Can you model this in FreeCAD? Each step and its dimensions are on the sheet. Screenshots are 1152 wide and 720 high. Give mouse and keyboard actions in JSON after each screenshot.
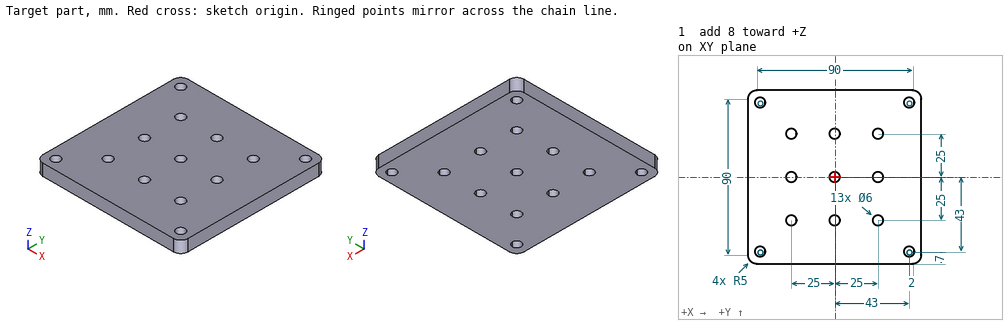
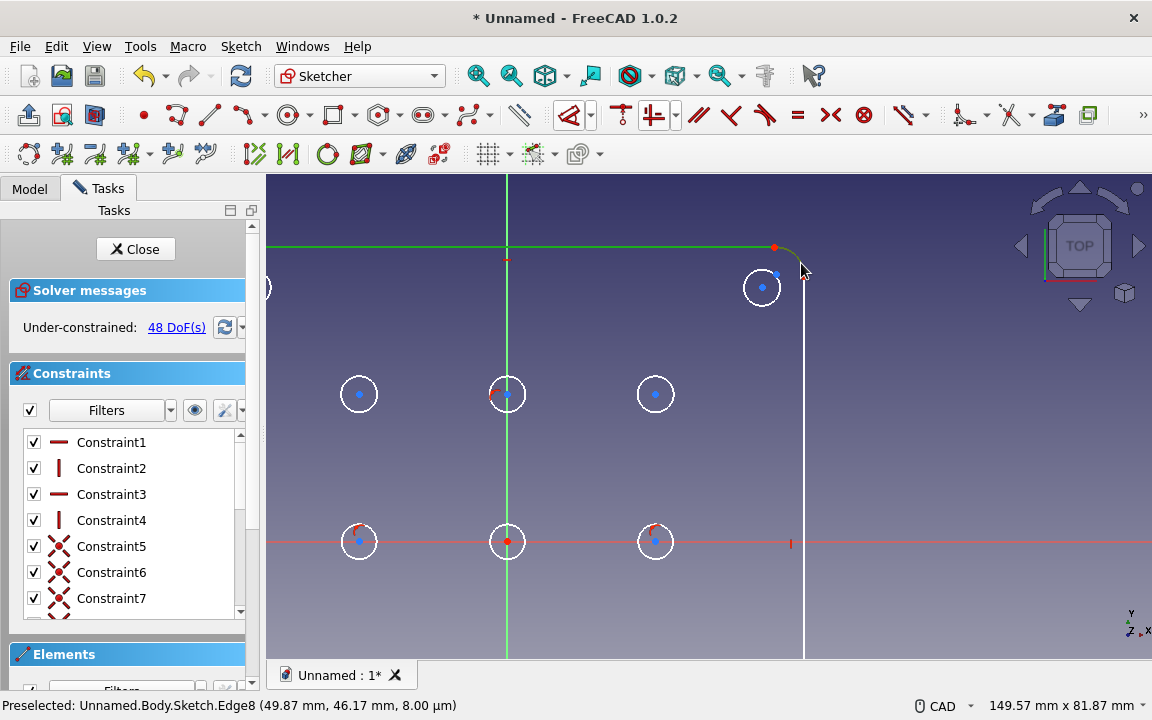
{"action": "left_click", "coordinate": [765, 116]}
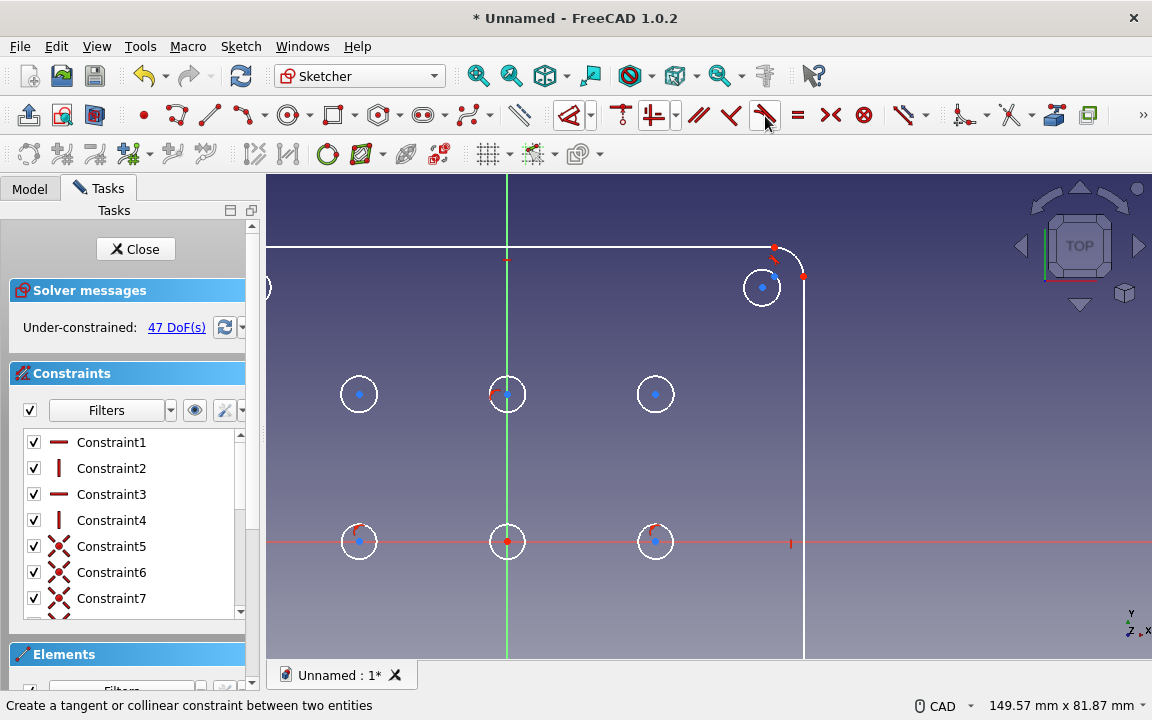
{"action": "scroll", "coordinate": [802, 264], "scroll_direction": "down", "scroll_amount": 3}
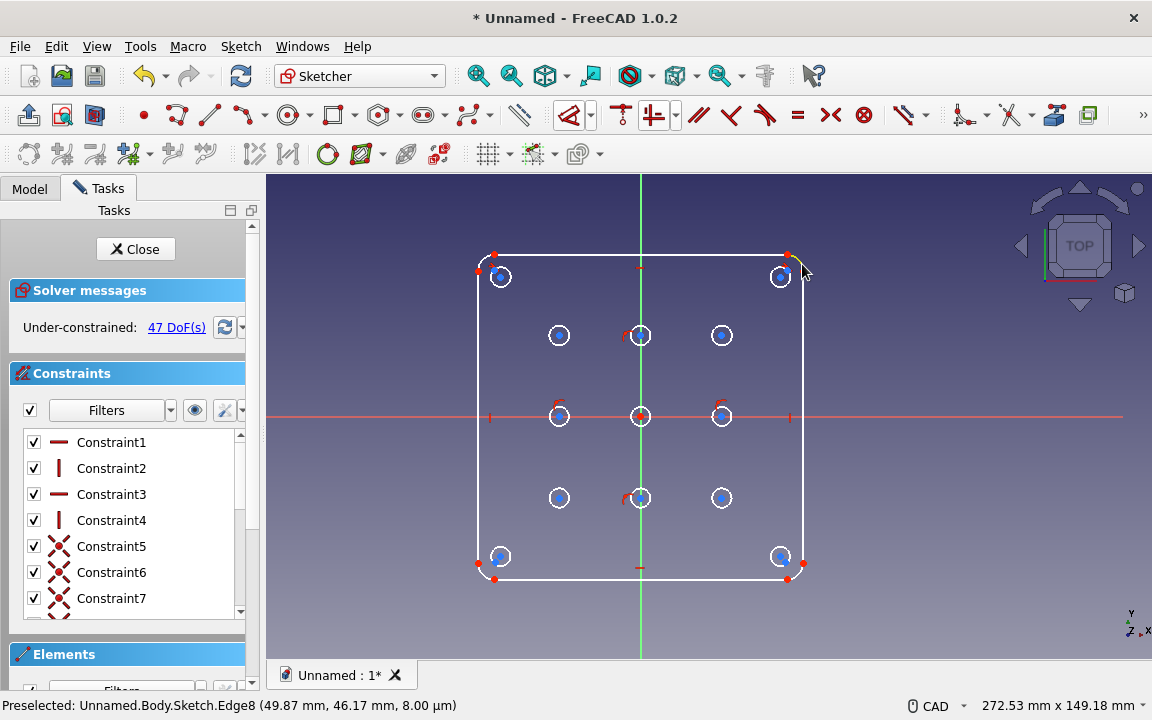
{"action": "left_click", "coordinate": [478, 359]}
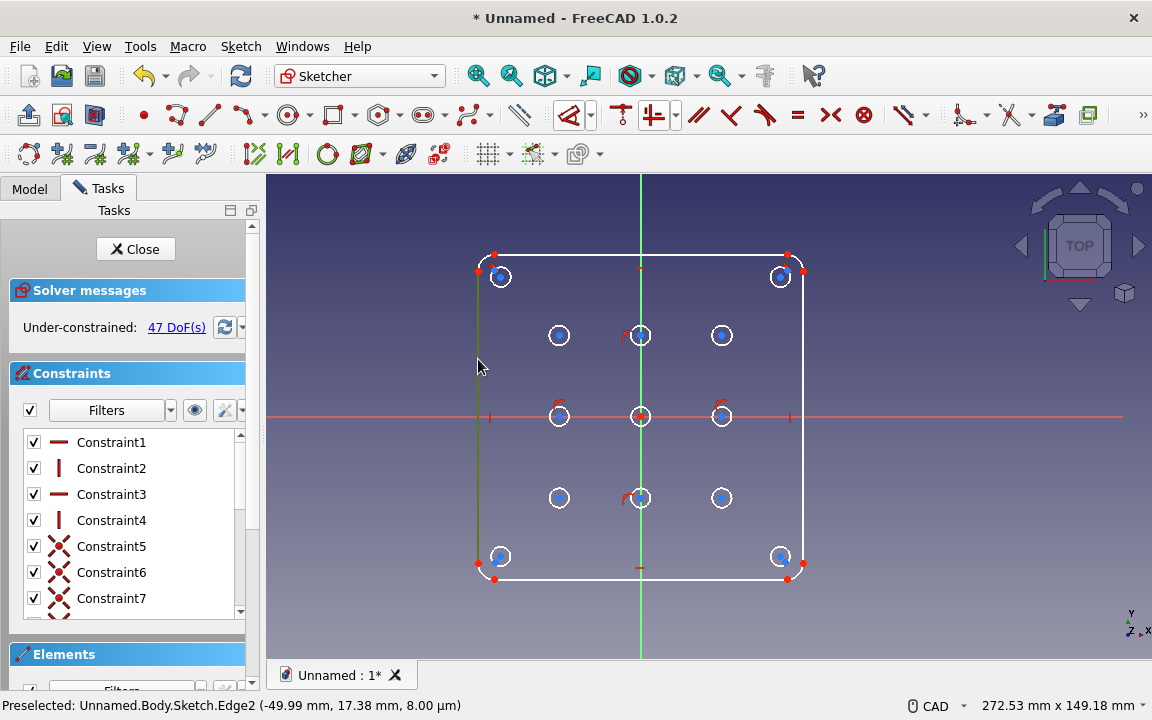
{"action": "left_click", "coordinate": [483, 260]}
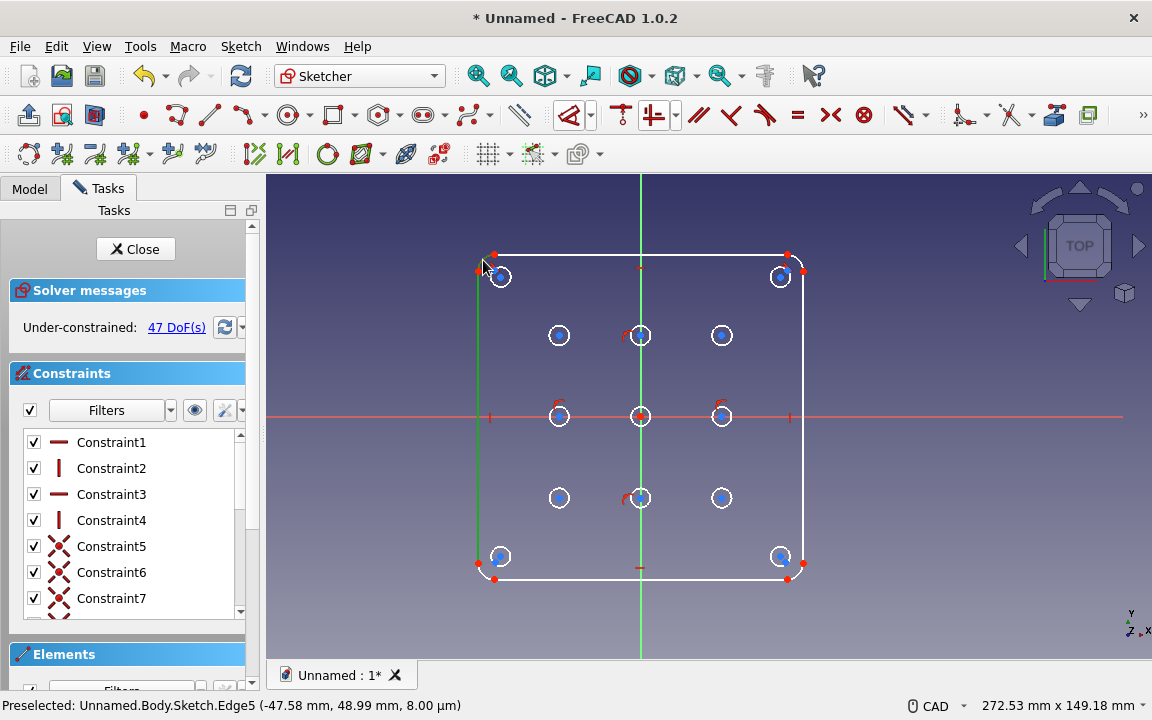
{"action": "left_click", "coordinate": [765, 116]}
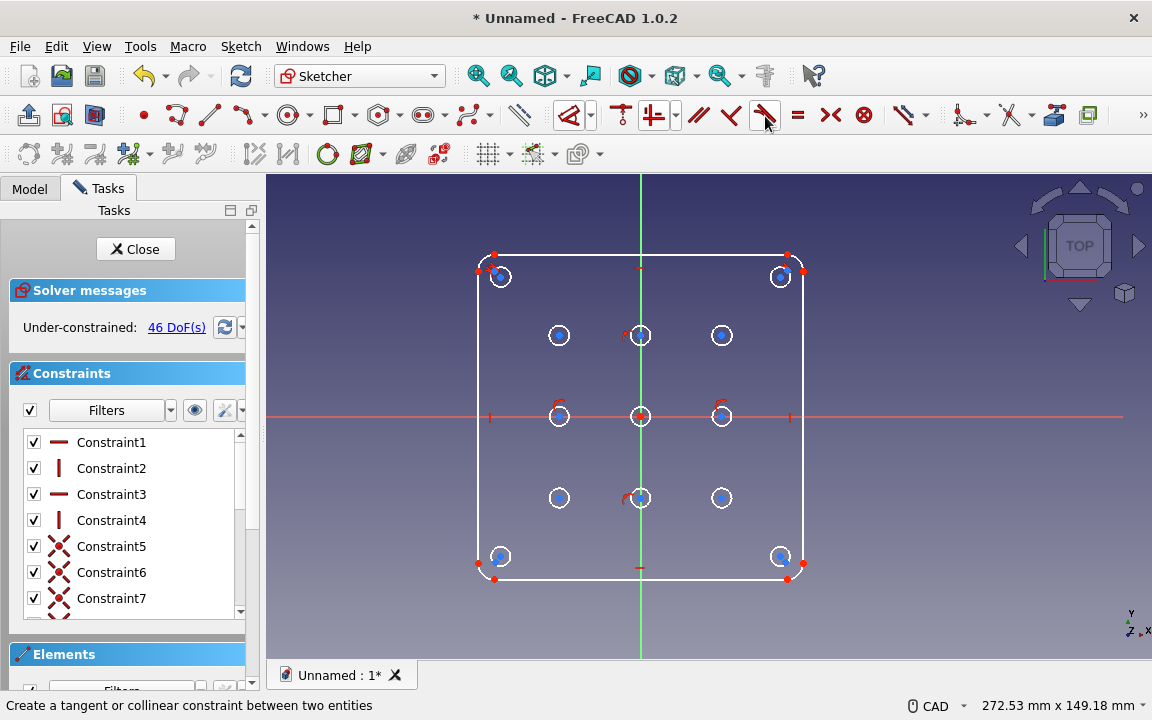
{"action": "left_click", "coordinate": [478, 359]}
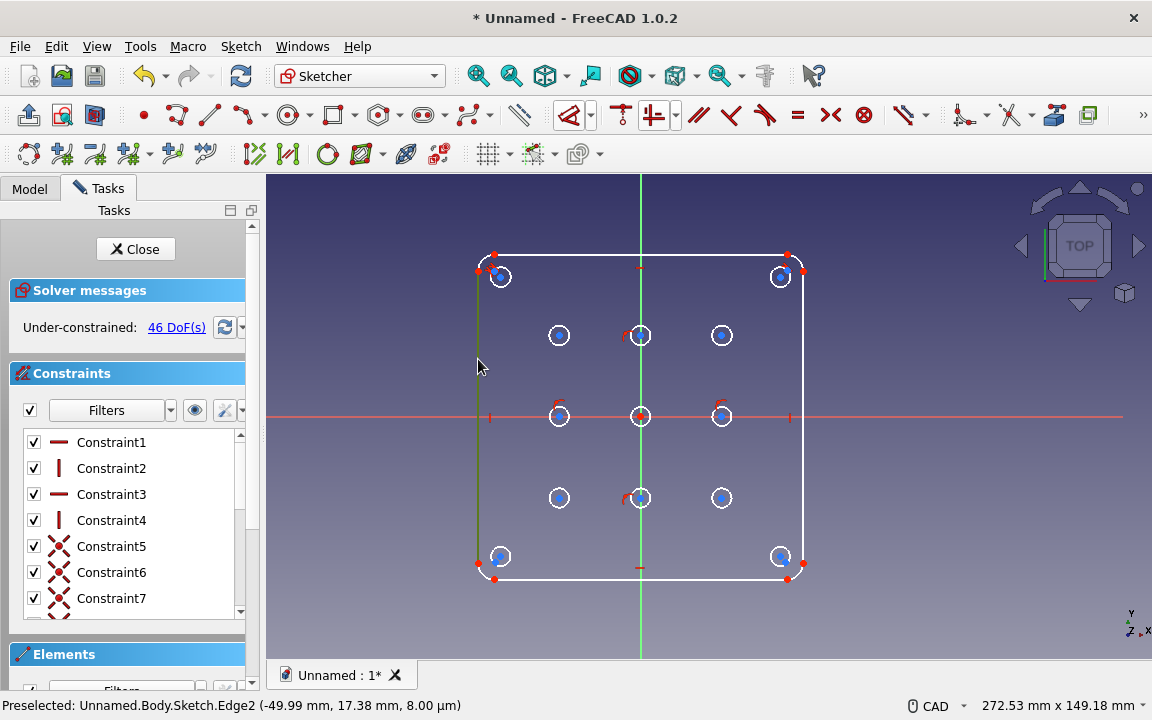
{"action": "left_click", "coordinate": [483, 575]}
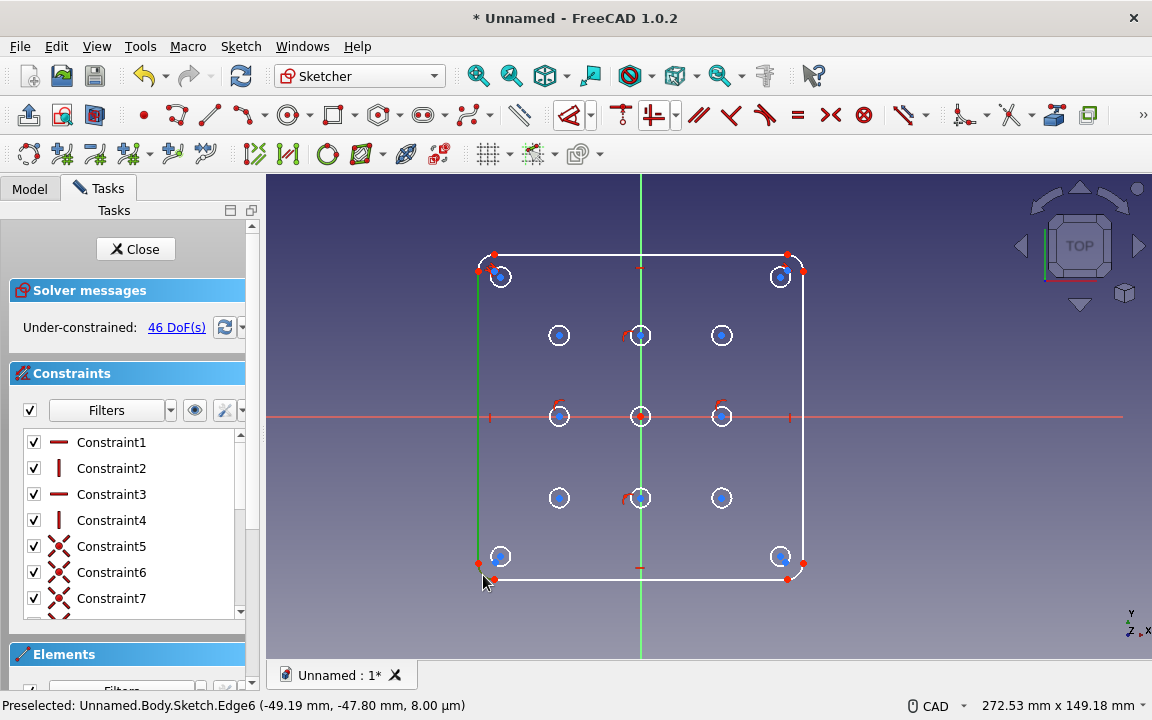
{"action": "left_click", "coordinate": [765, 116]}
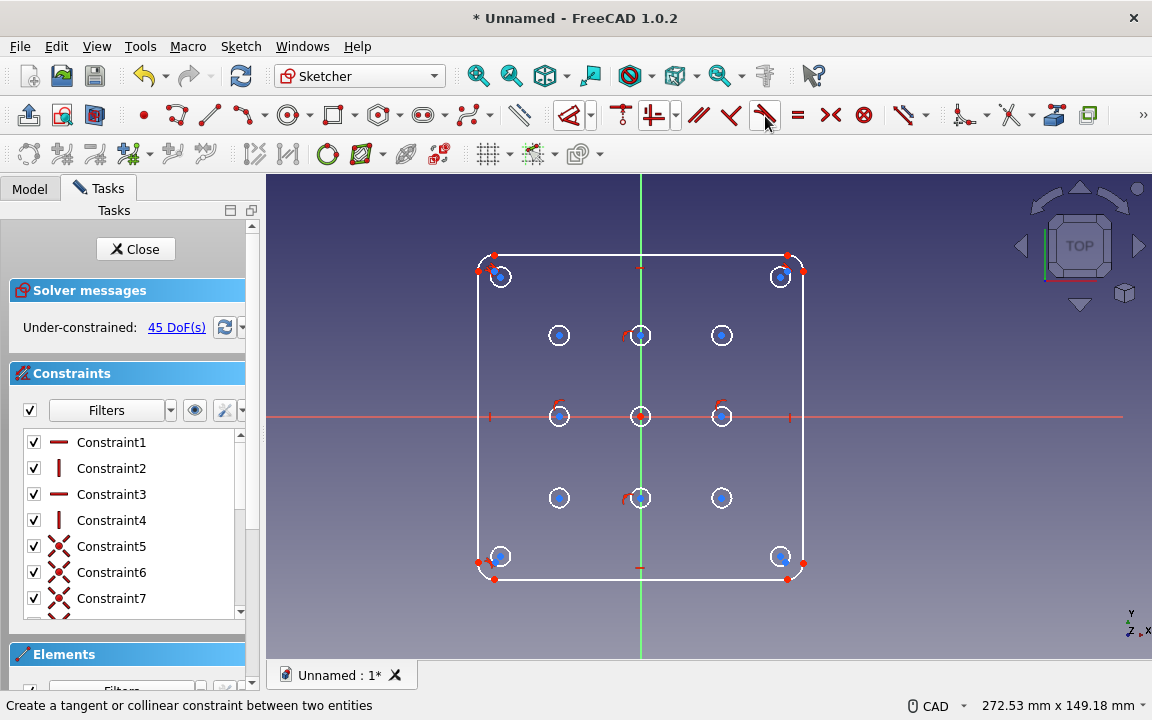
{"action": "left_click", "coordinate": [582, 580]}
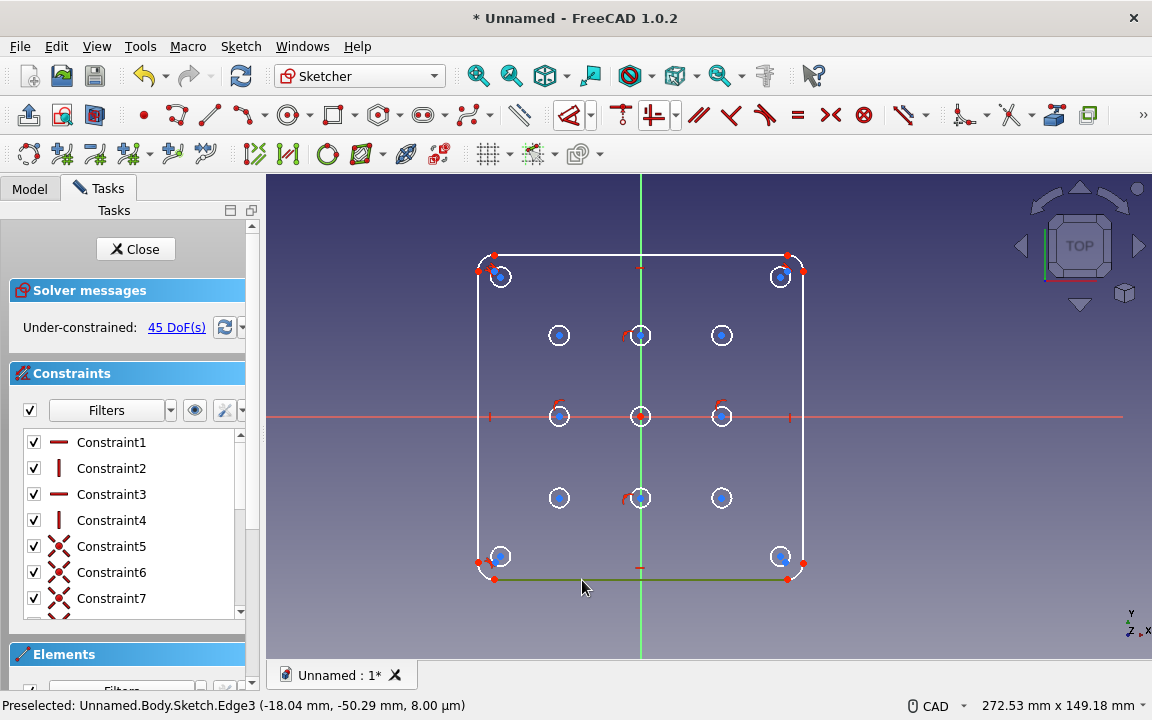
{"action": "left_click", "coordinate": [483, 575]}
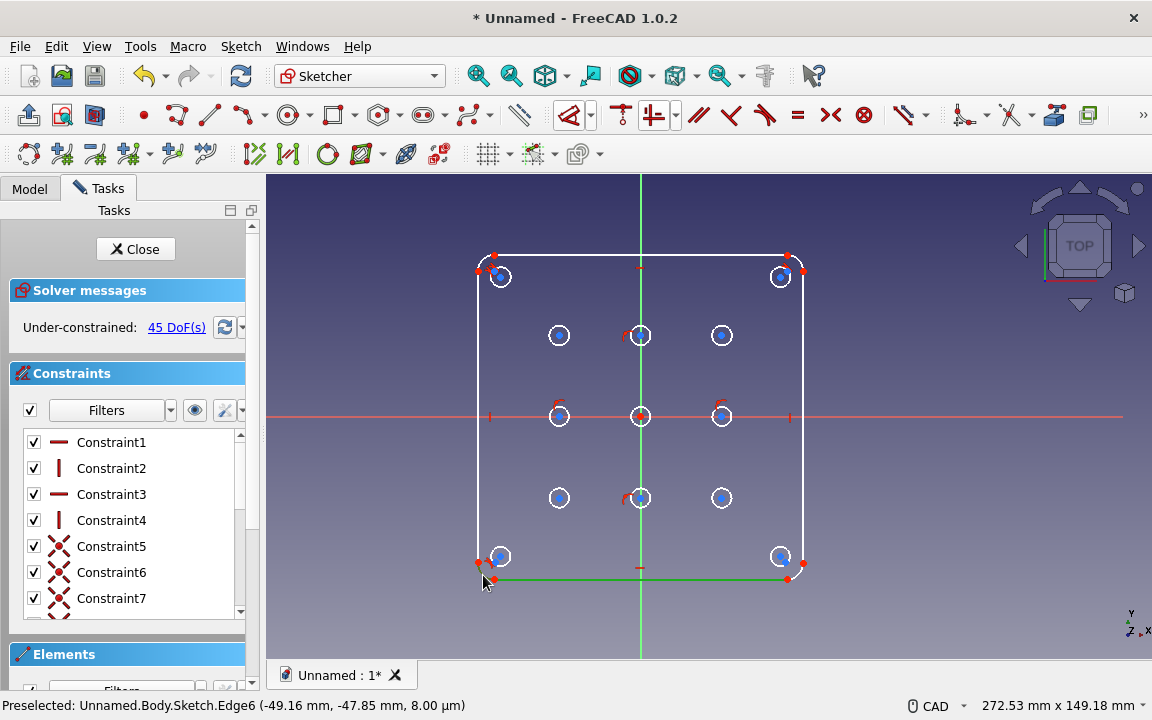
{"action": "left_click", "coordinate": [765, 116]}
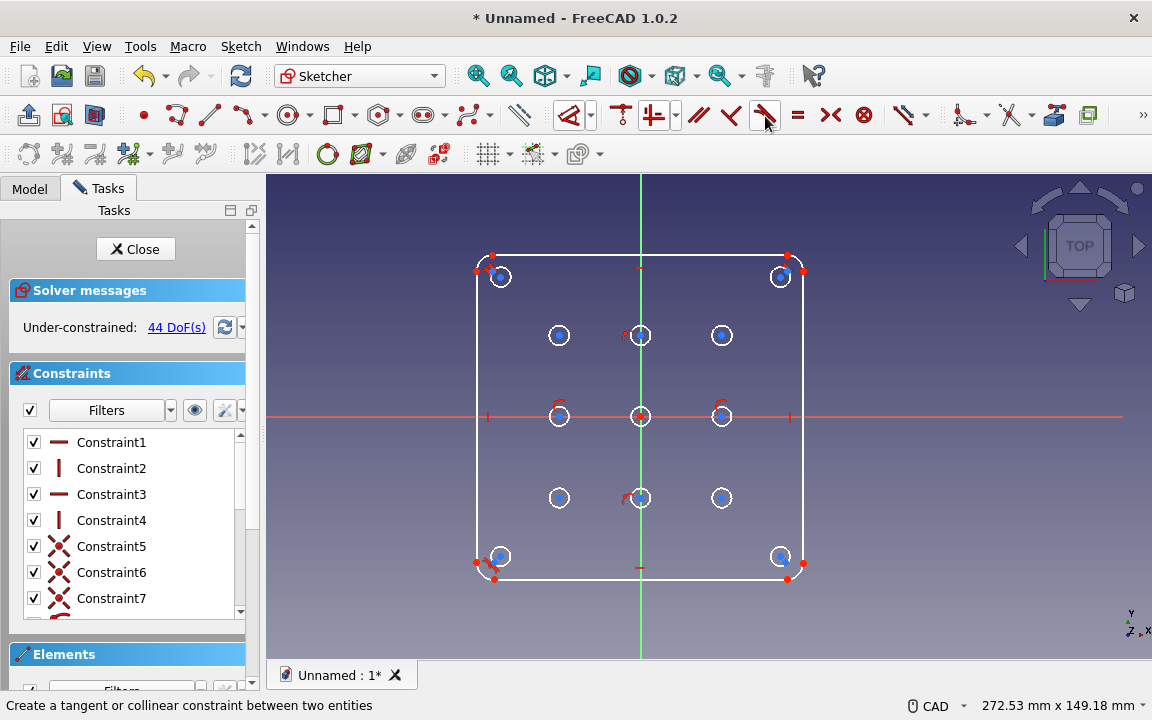
{"action": "left_click", "coordinate": [582, 580]}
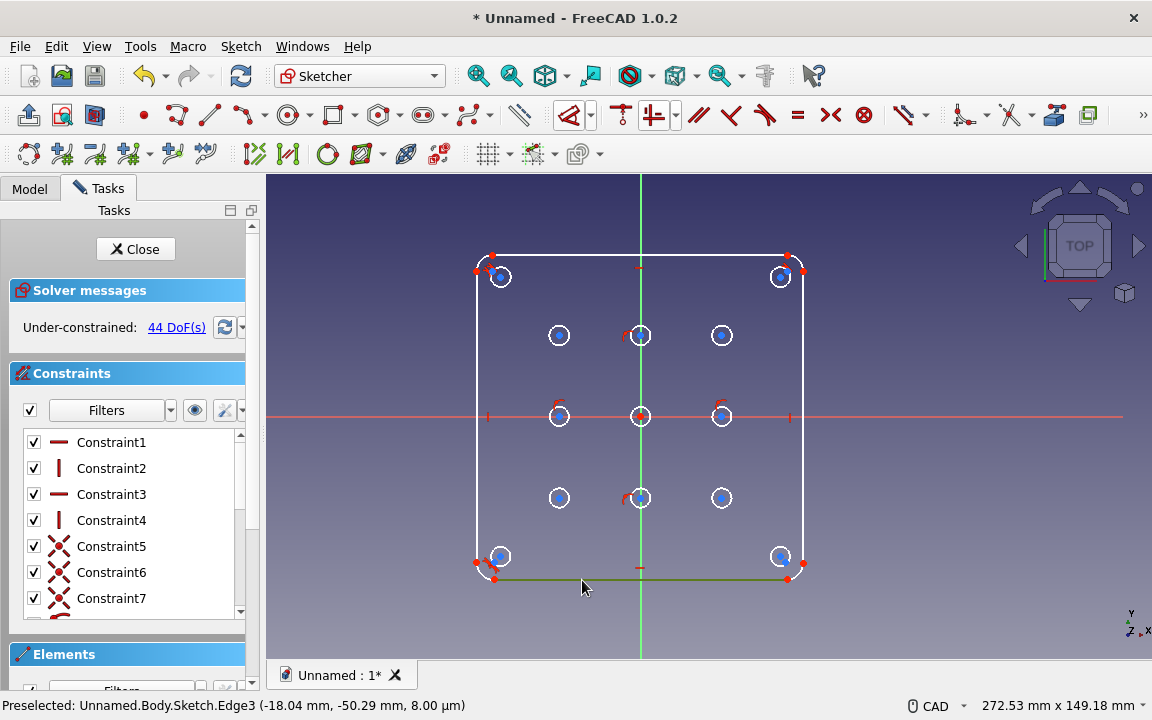
{"action": "left_click", "coordinate": [798, 575]}